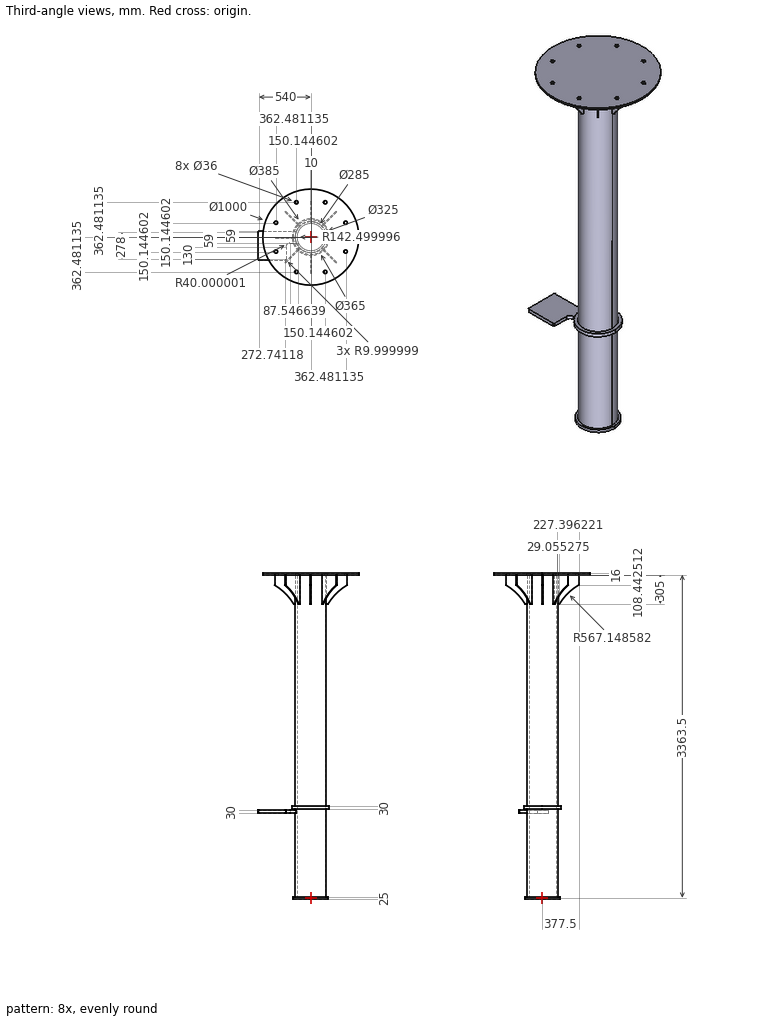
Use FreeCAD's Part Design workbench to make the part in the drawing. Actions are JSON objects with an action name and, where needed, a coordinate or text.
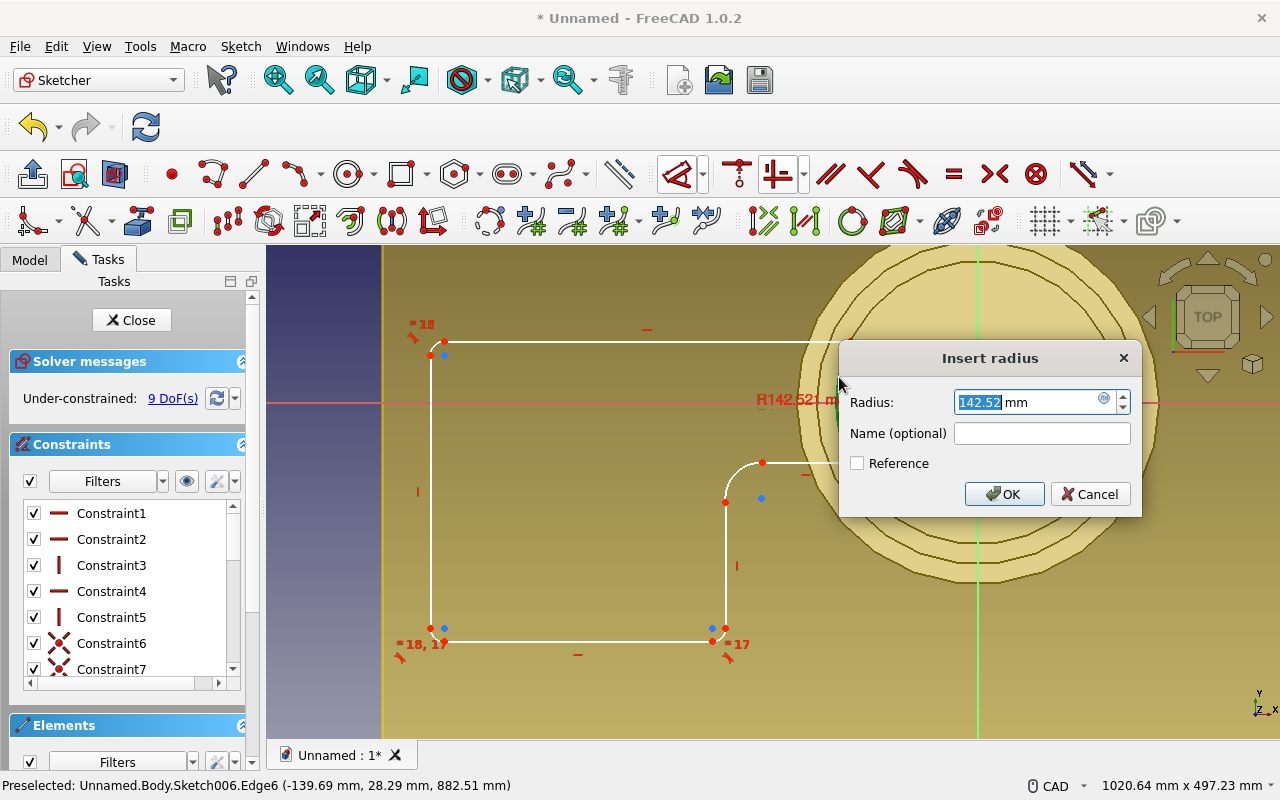
{"action": "type", "text": "142.499996"}
{"action": "key", "text": "Return"}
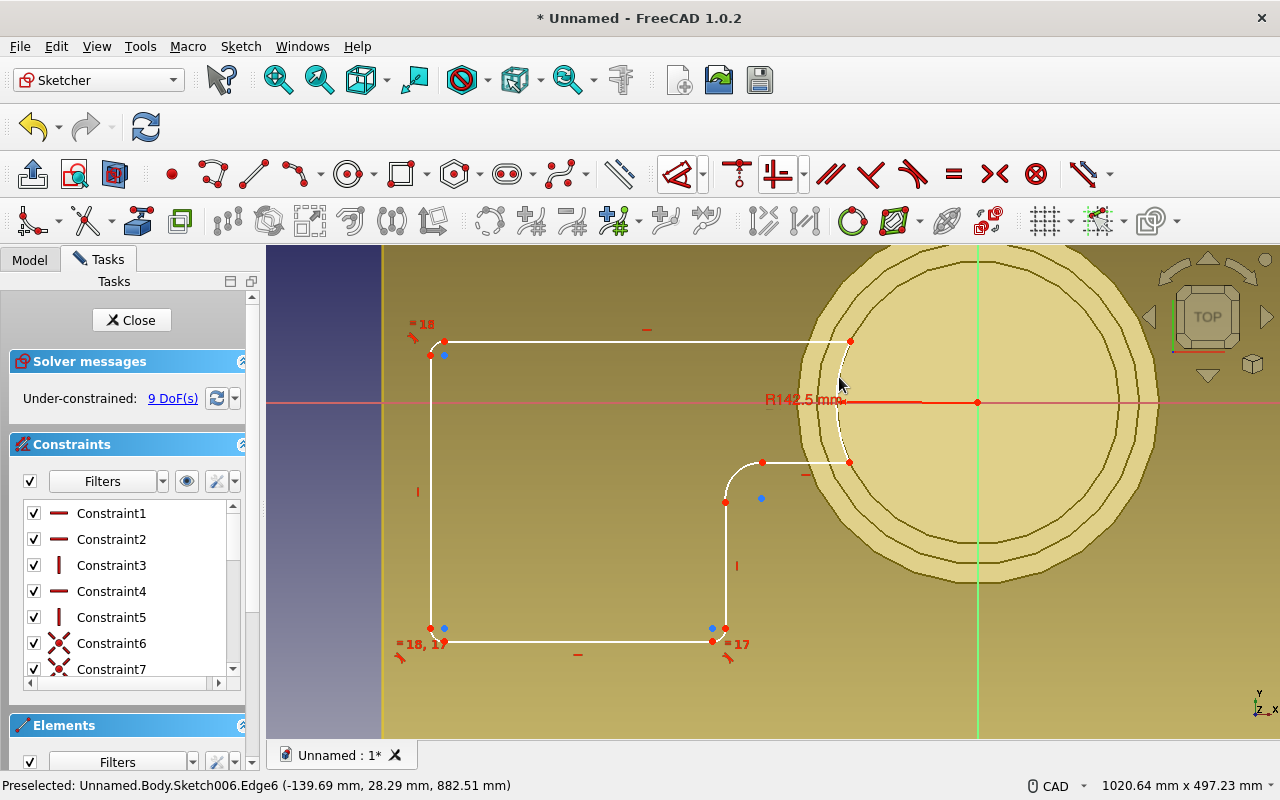
{"action": "left_click", "coordinate": [745, 467]}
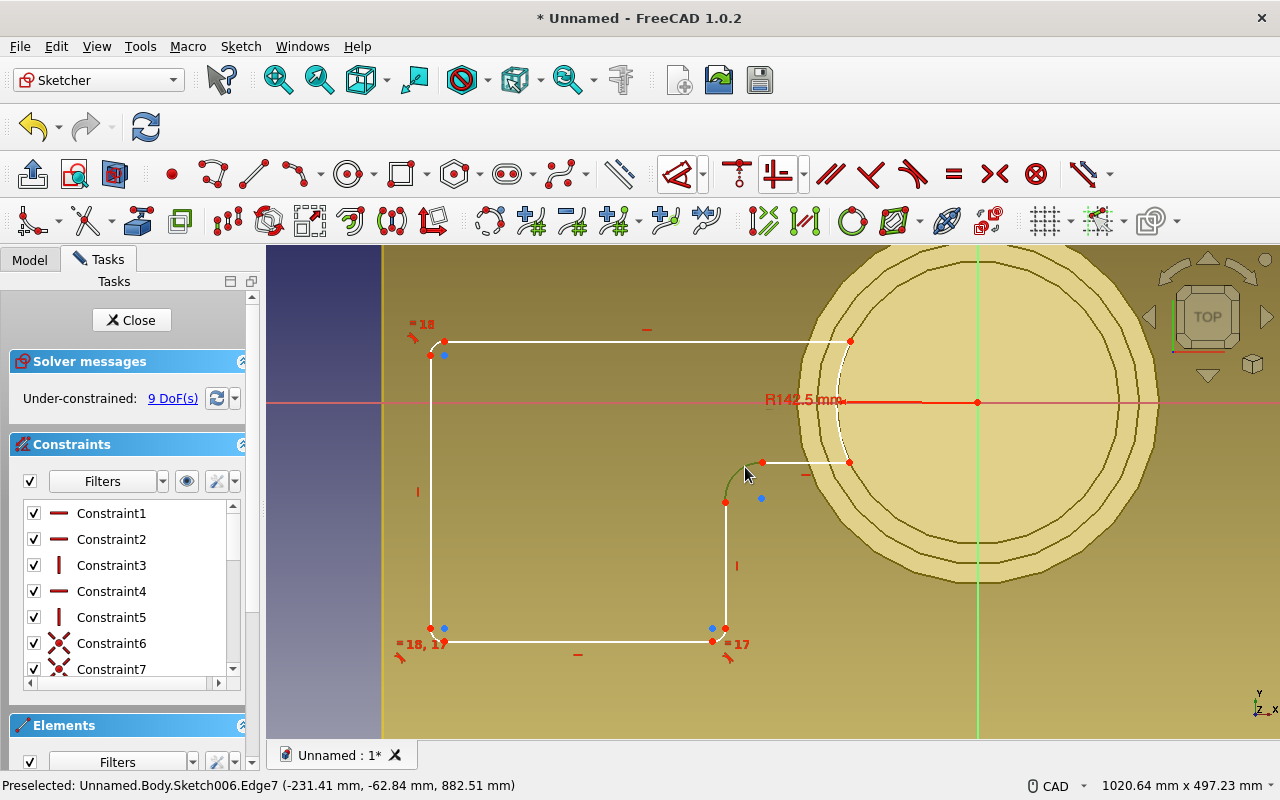
{"action": "key", "text": "k r"}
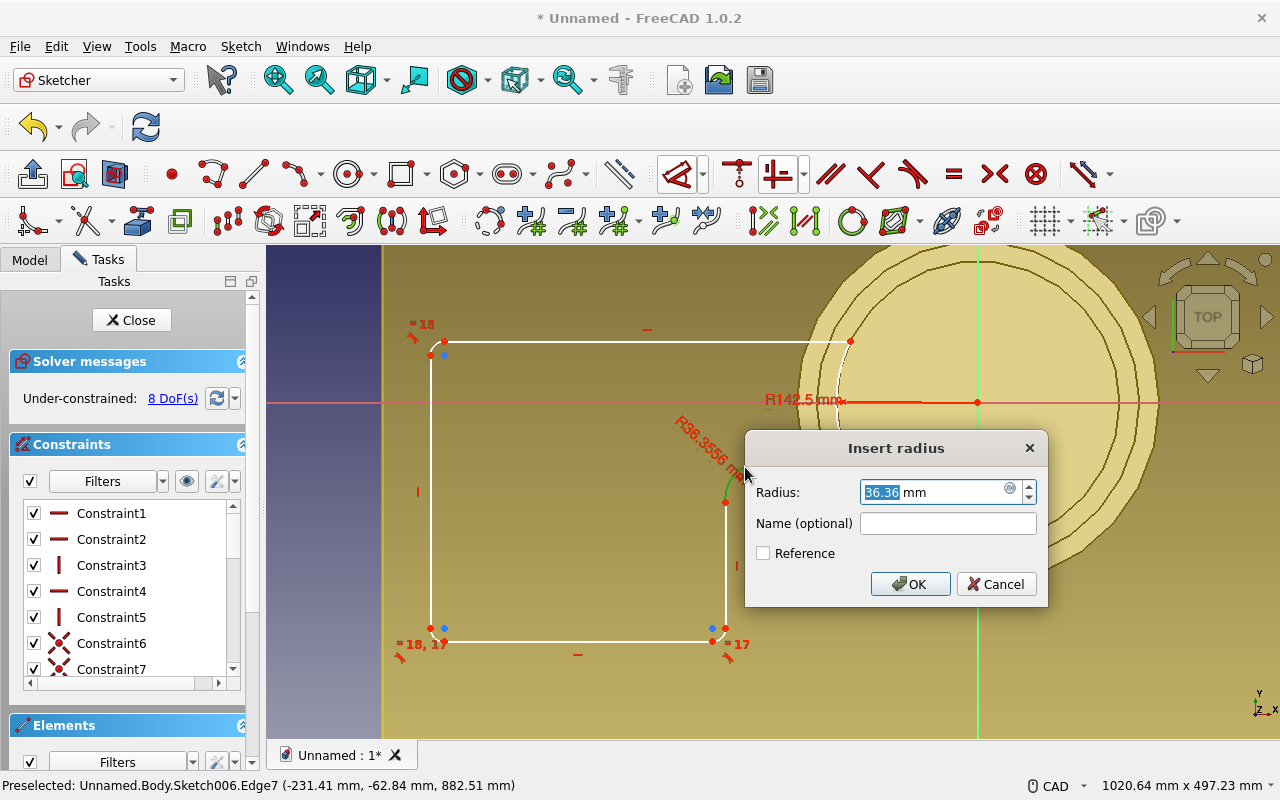
{"action": "type", "text": "40.000001"}
{"action": "key", "text": "Return"}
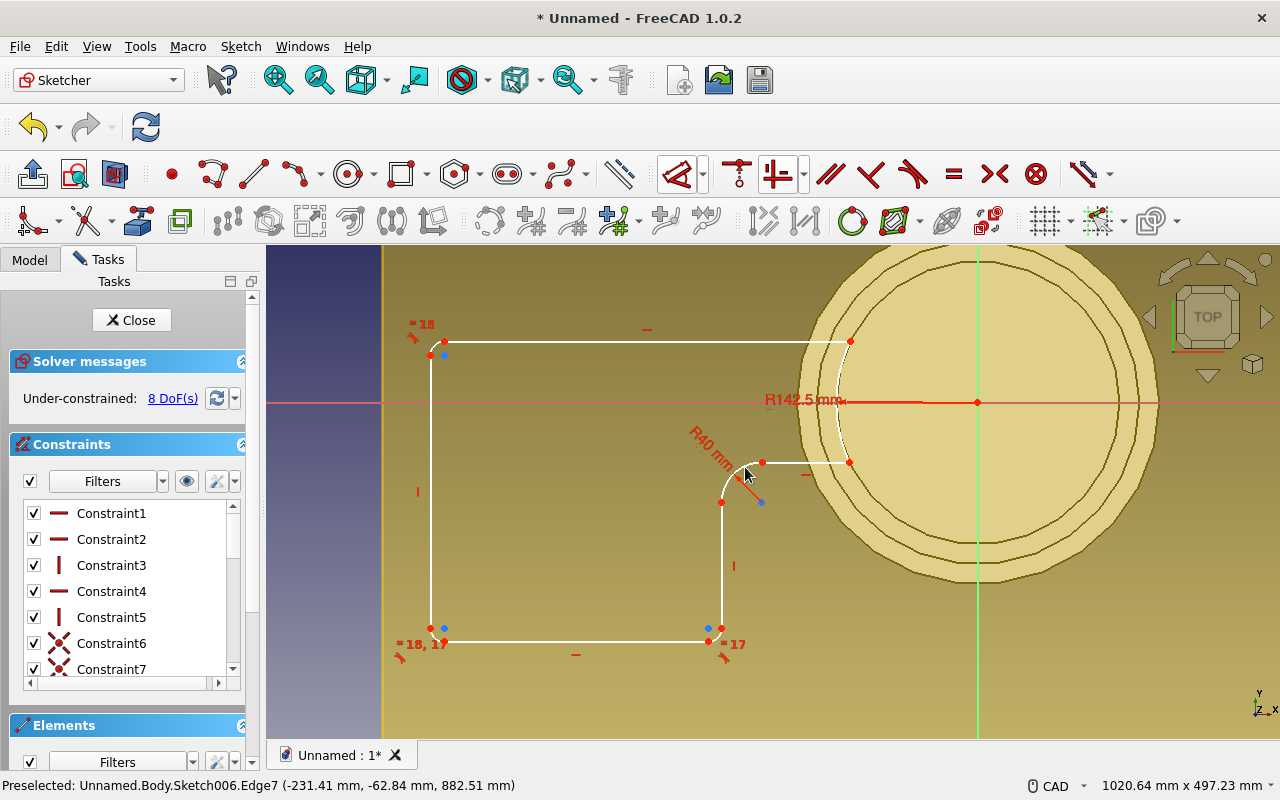
{"action": "scroll", "coordinate": [718, 638], "scroll_direction": "up", "scroll_amount": 7}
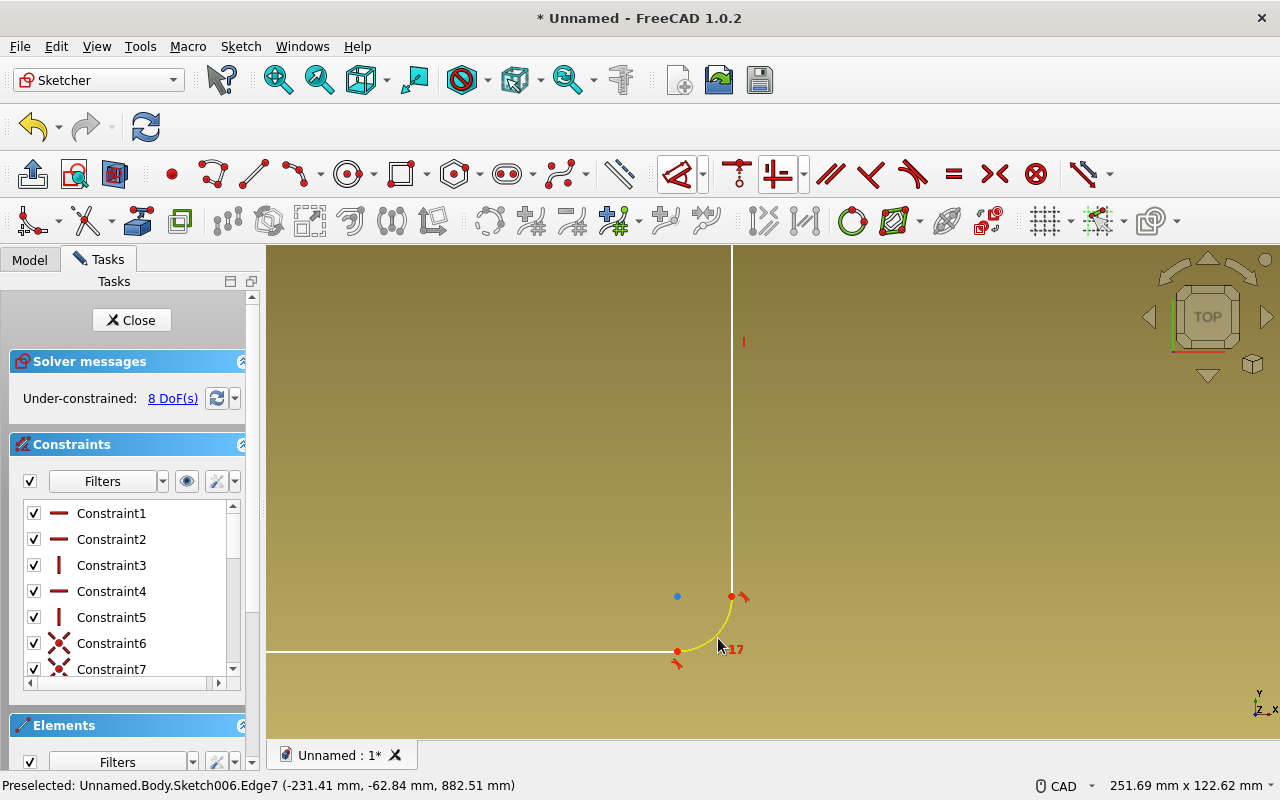
{"action": "left_click", "coordinate": [716, 636]}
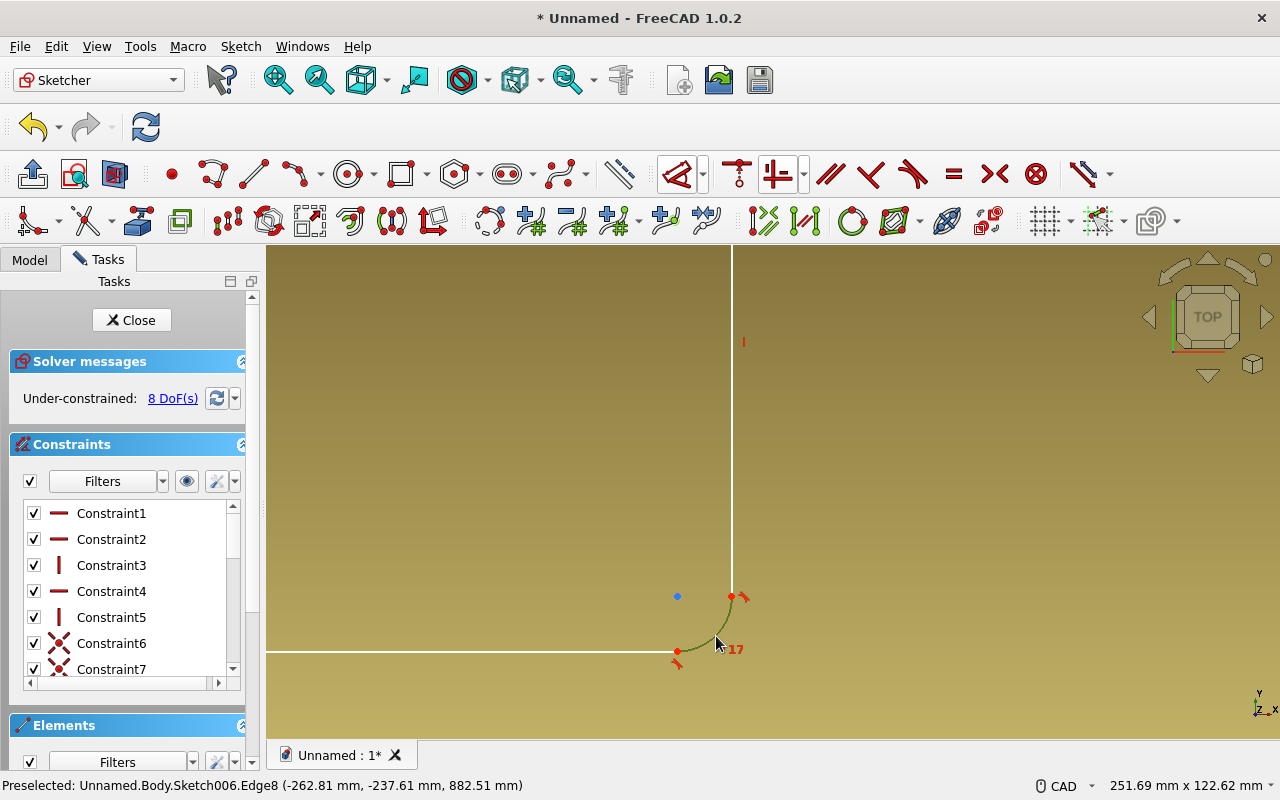
{"action": "key", "text": "k r"}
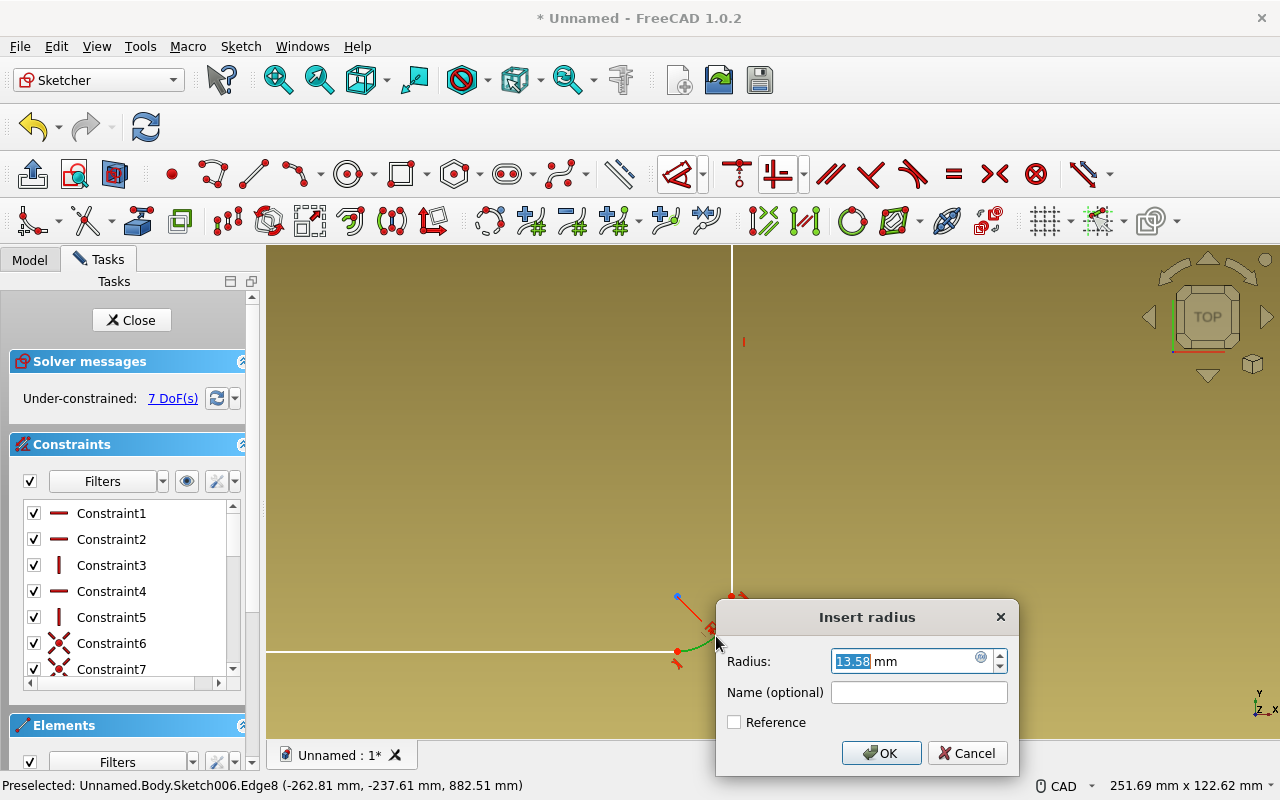
{"action": "type", "text": "9.999999"}
{"action": "key", "text": "Return"}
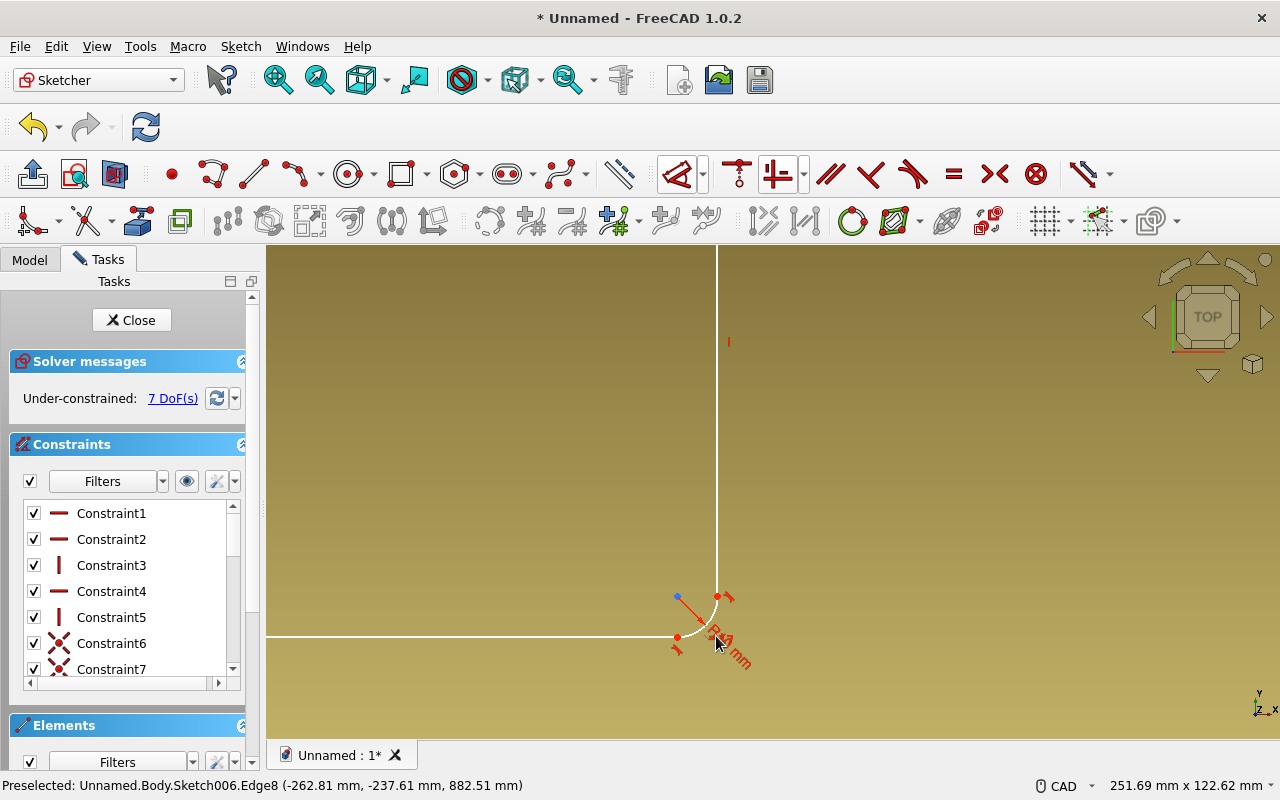
{"action": "scroll", "coordinate": [718, 639], "scroll_direction": "down", "scroll_amount": 7}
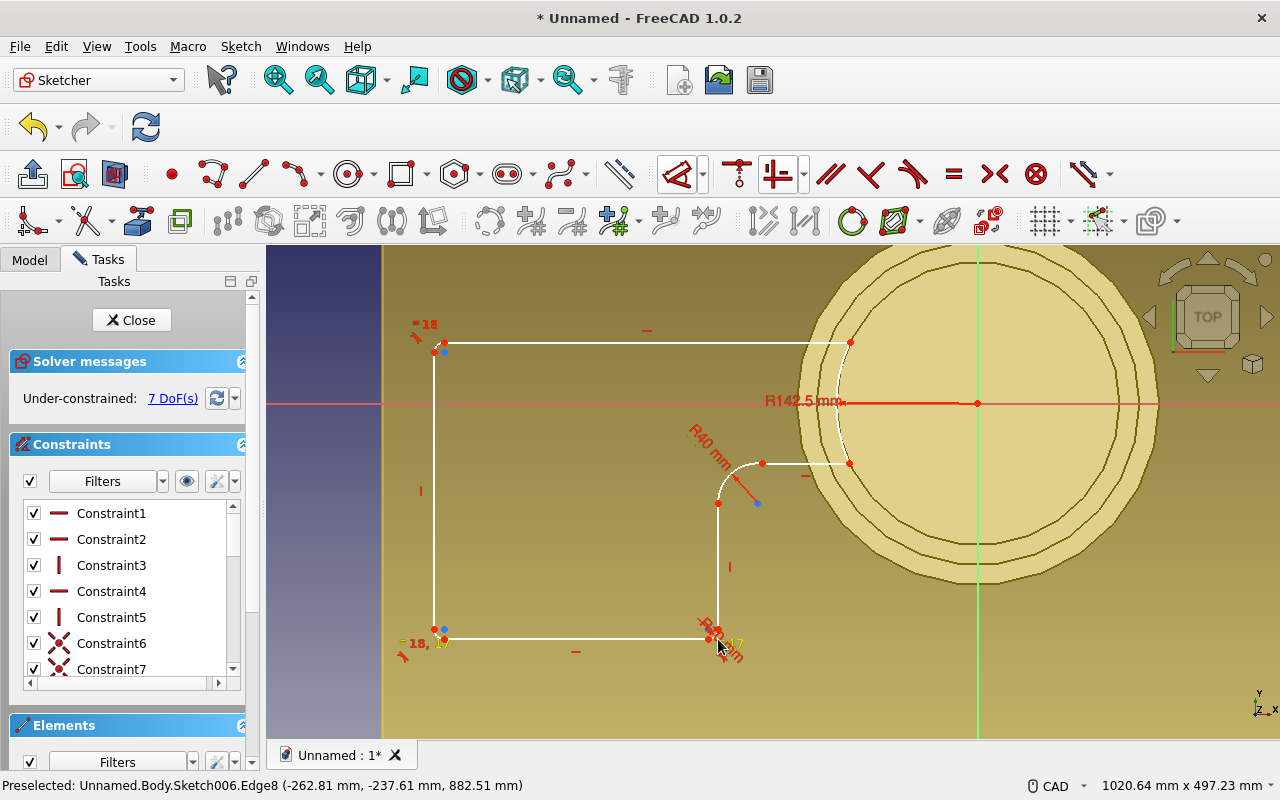
{"action": "left_click", "coordinate": [718, 591]}